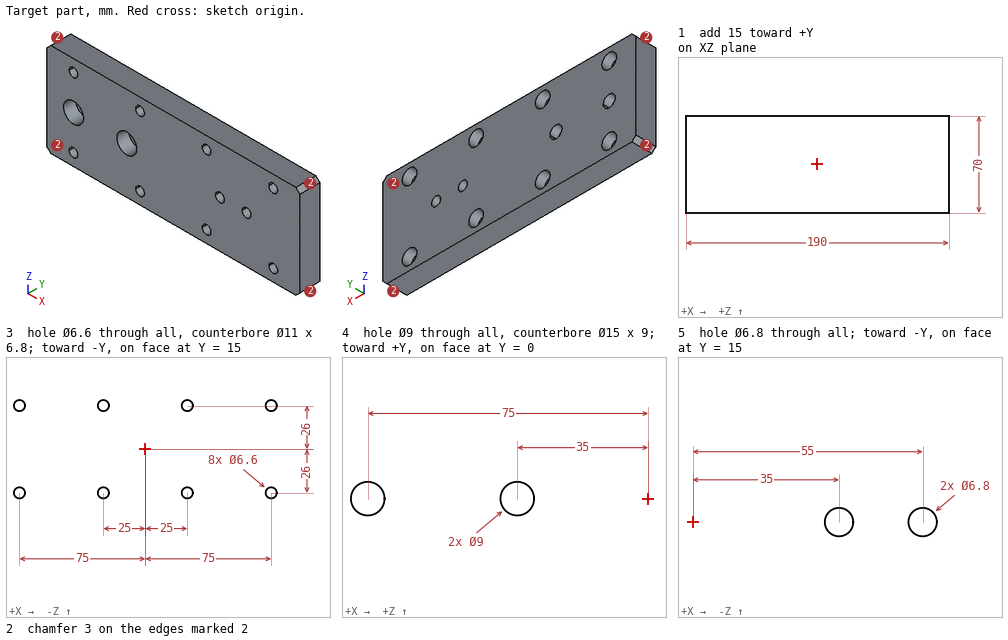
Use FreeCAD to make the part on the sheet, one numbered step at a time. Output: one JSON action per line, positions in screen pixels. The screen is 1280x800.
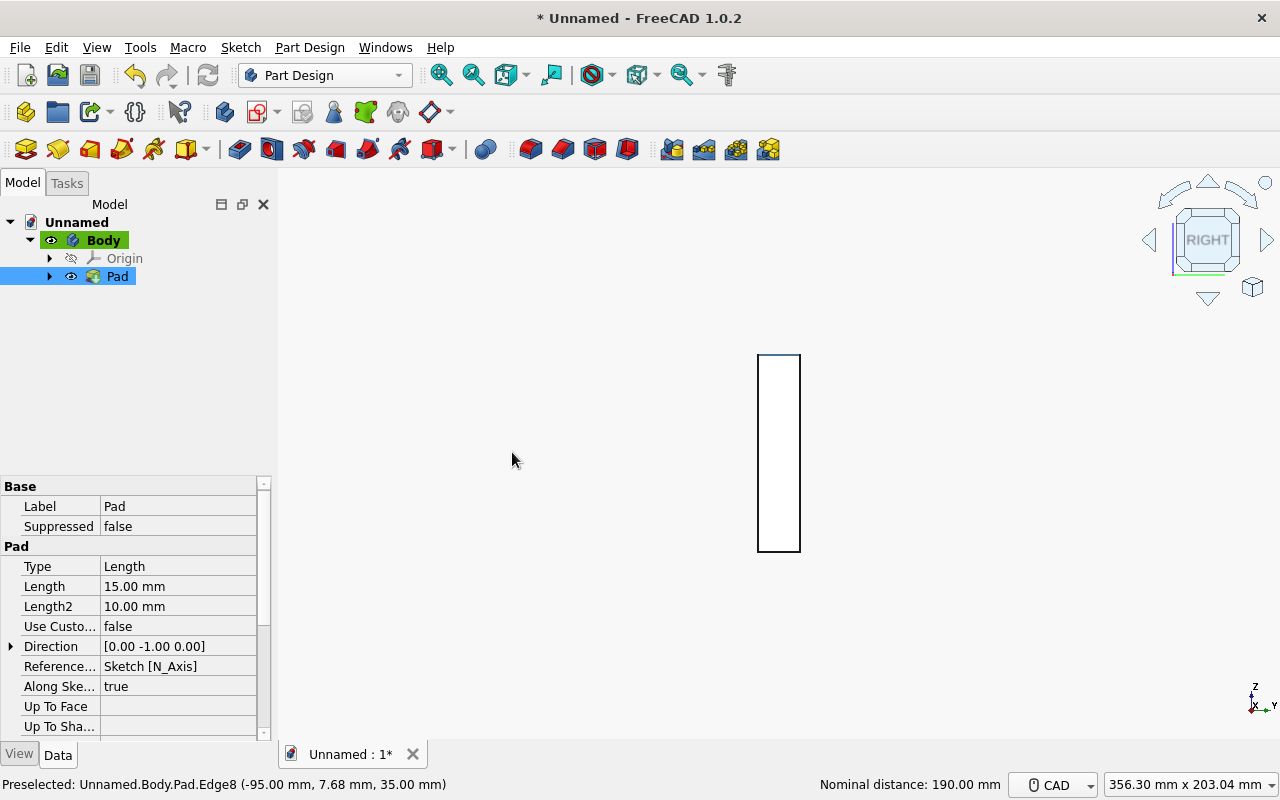
{"action": "key", "text": "v f"}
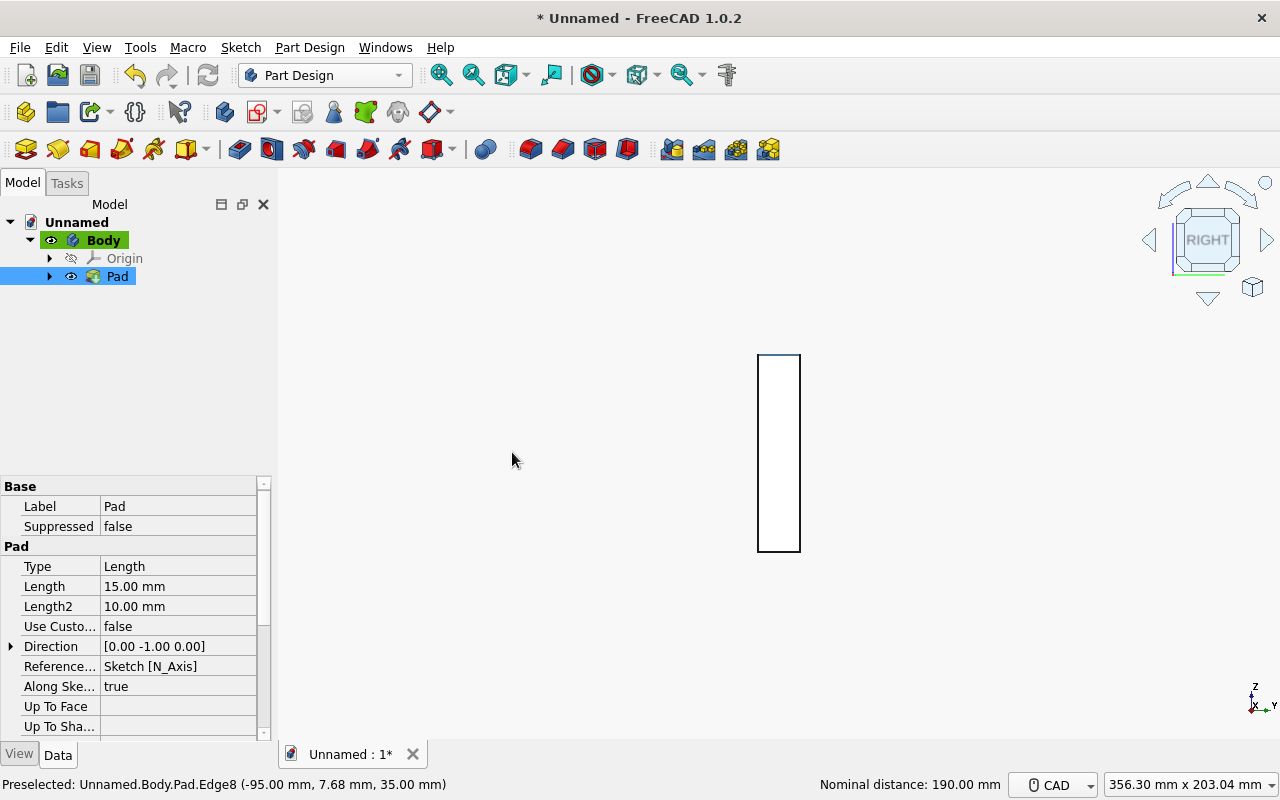
{"action": "left_click", "coordinate": [779, 551], "text": "ctrl"}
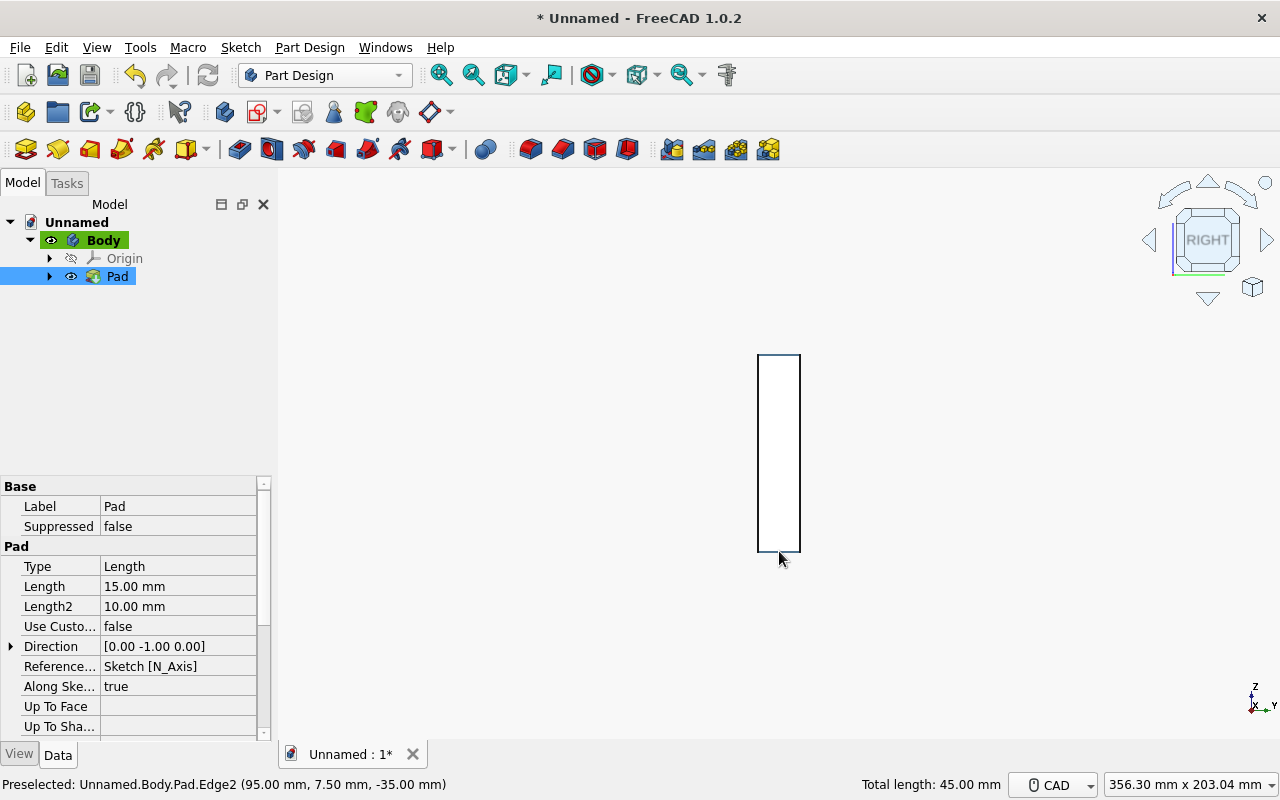
{"action": "key", "text": "5"}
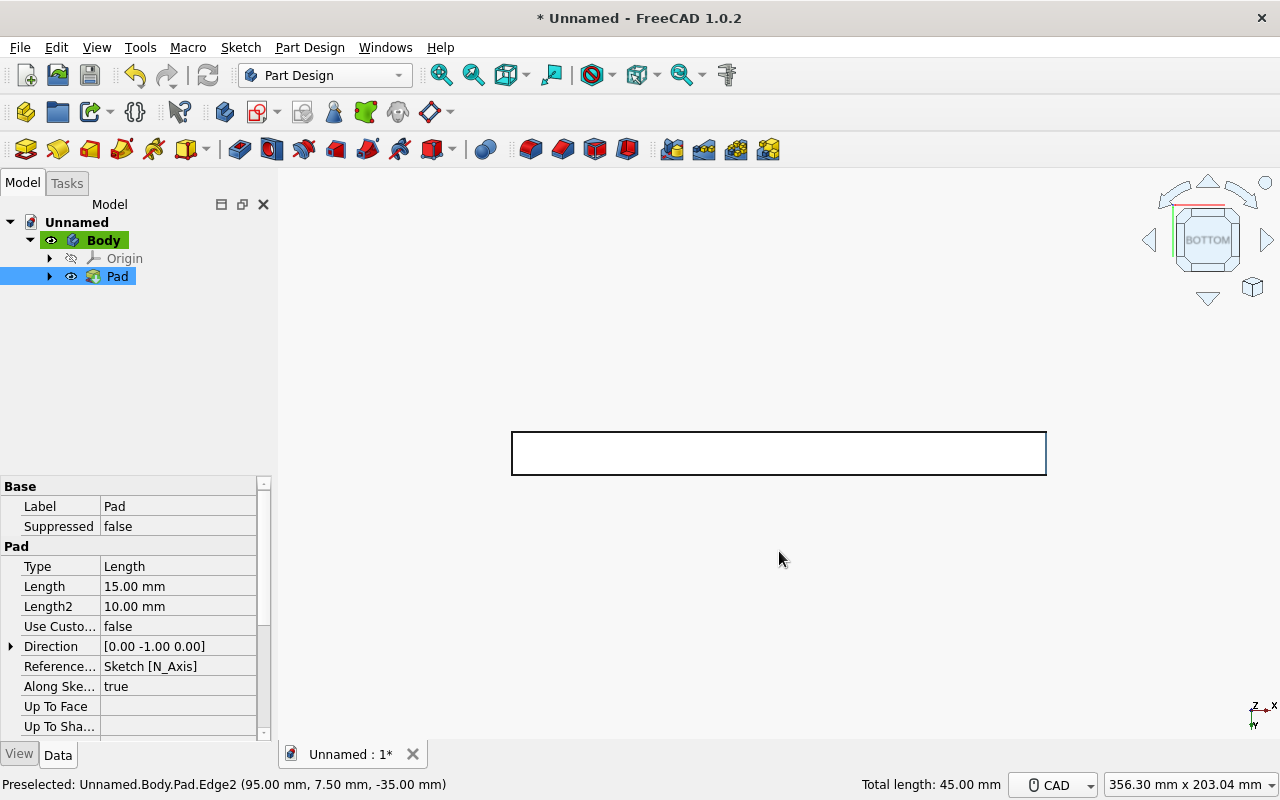
{"action": "left_click", "coordinate": [512, 452], "text": "ctrl"}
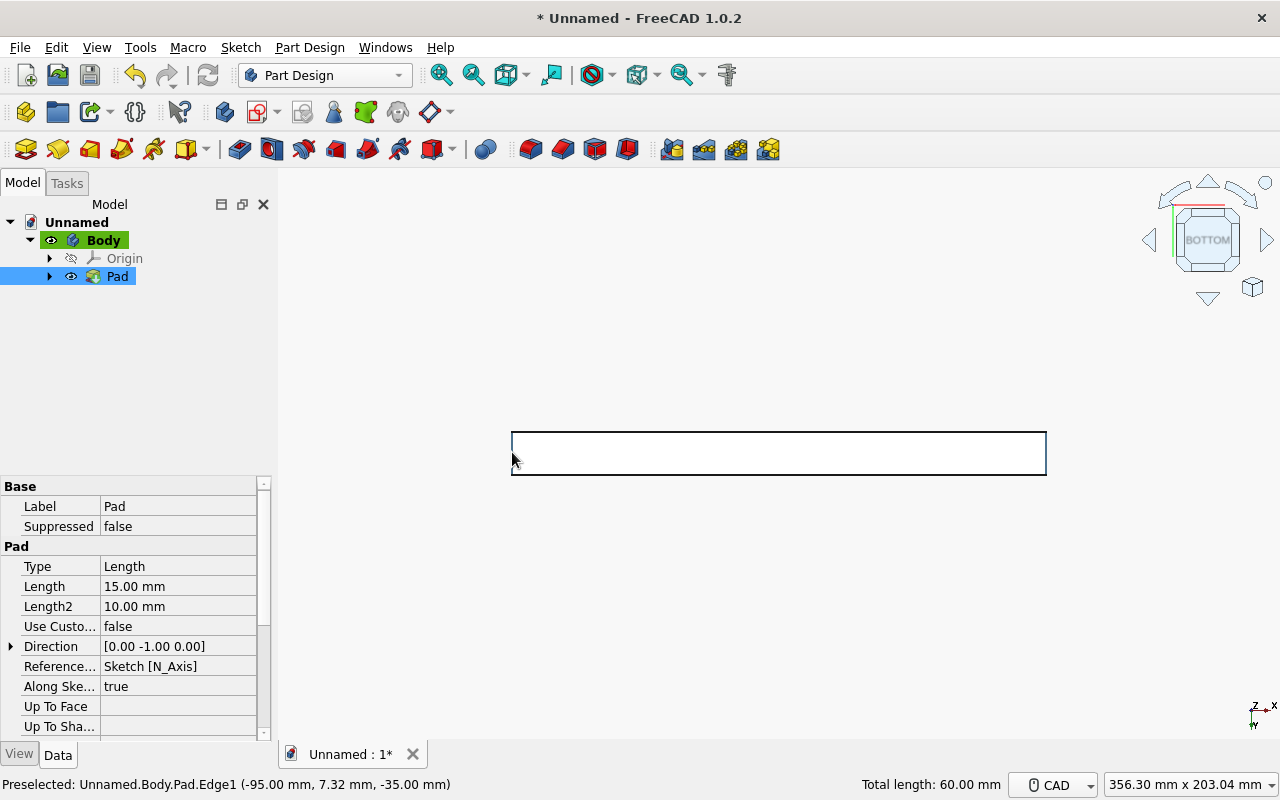
{"action": "left_click", "coordinate": [564, 150]}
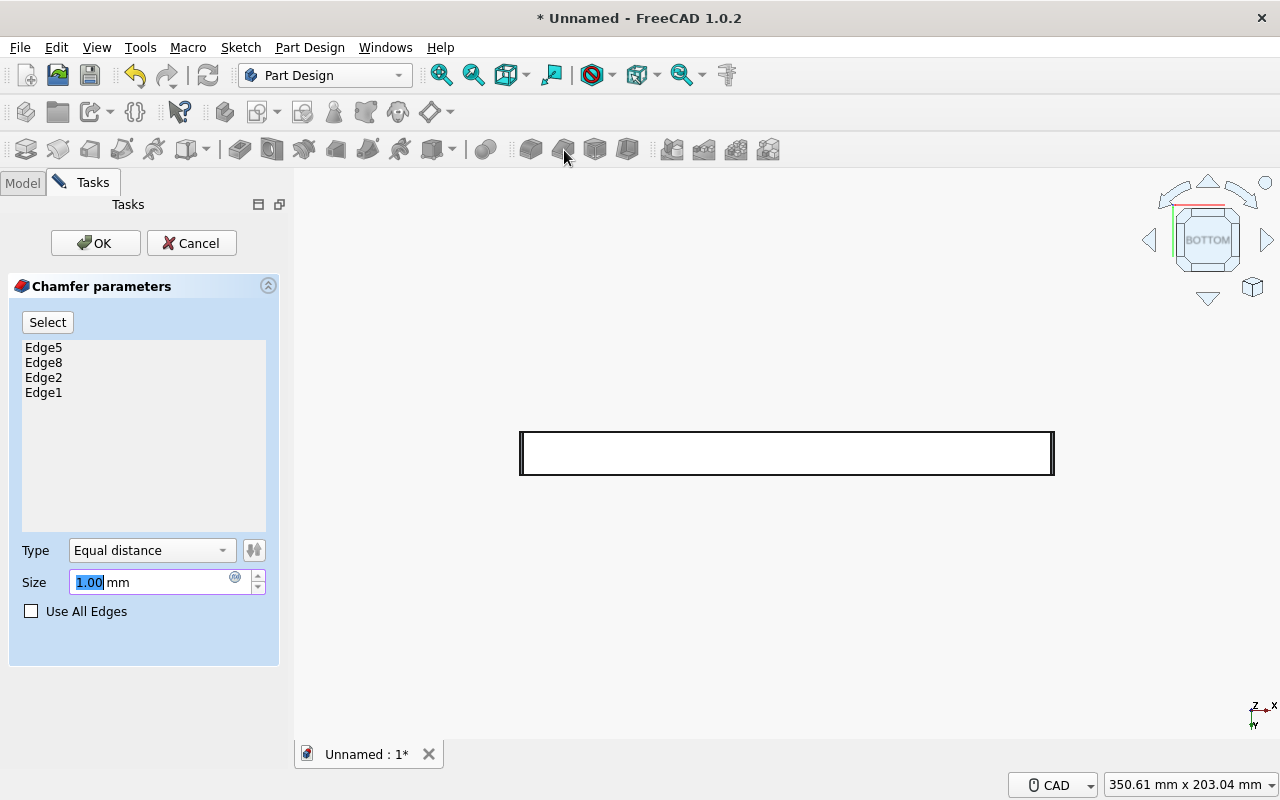
{"action": "type", "text": "3"}
{"action": "key", "text": "Tab"}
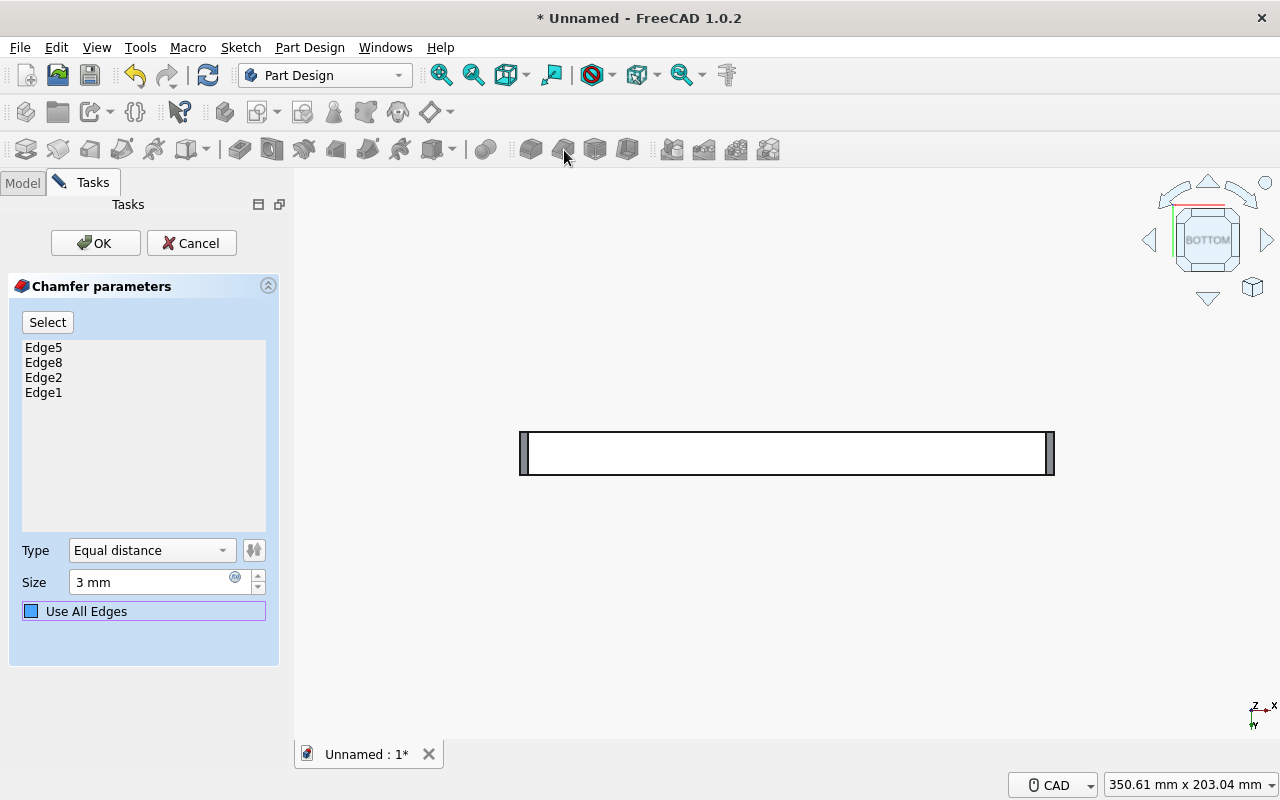
{"action": "left_click", "coordinate": [96, 243]}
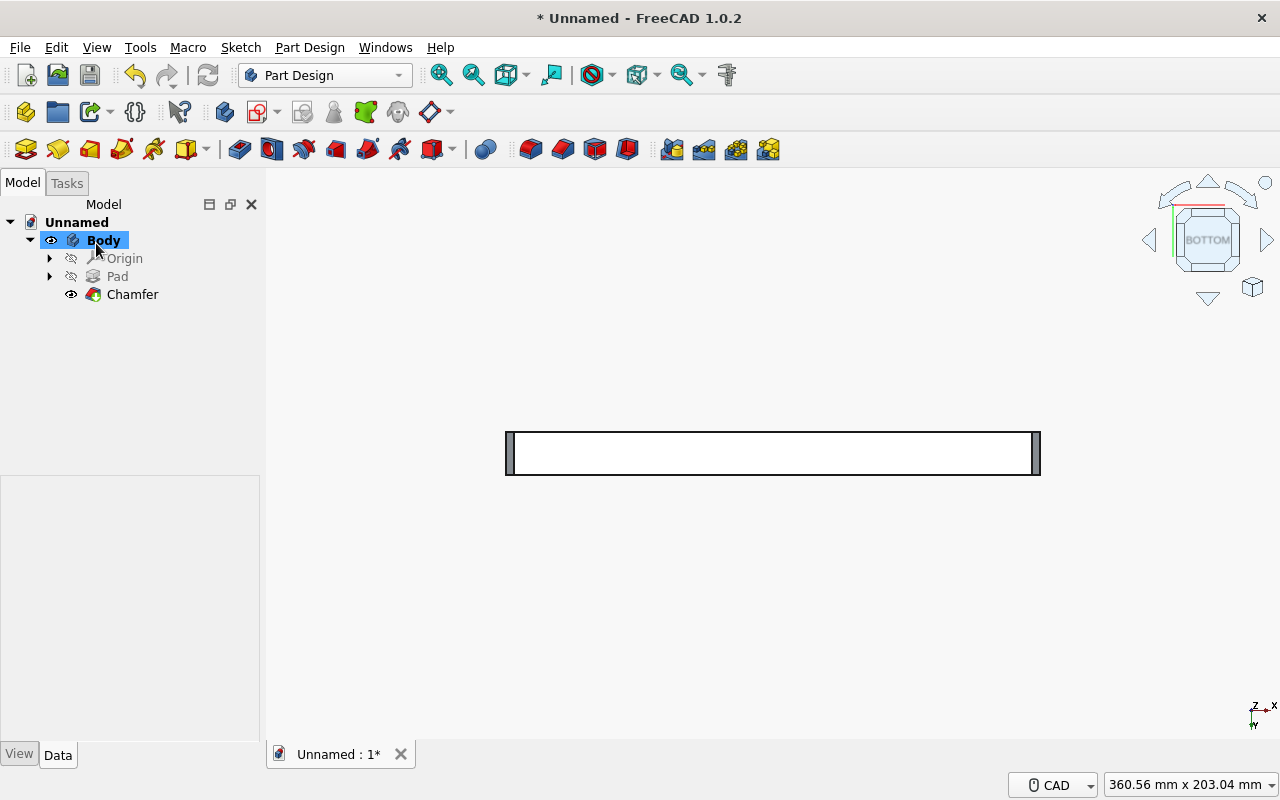
{"action": "key", "text": "4"}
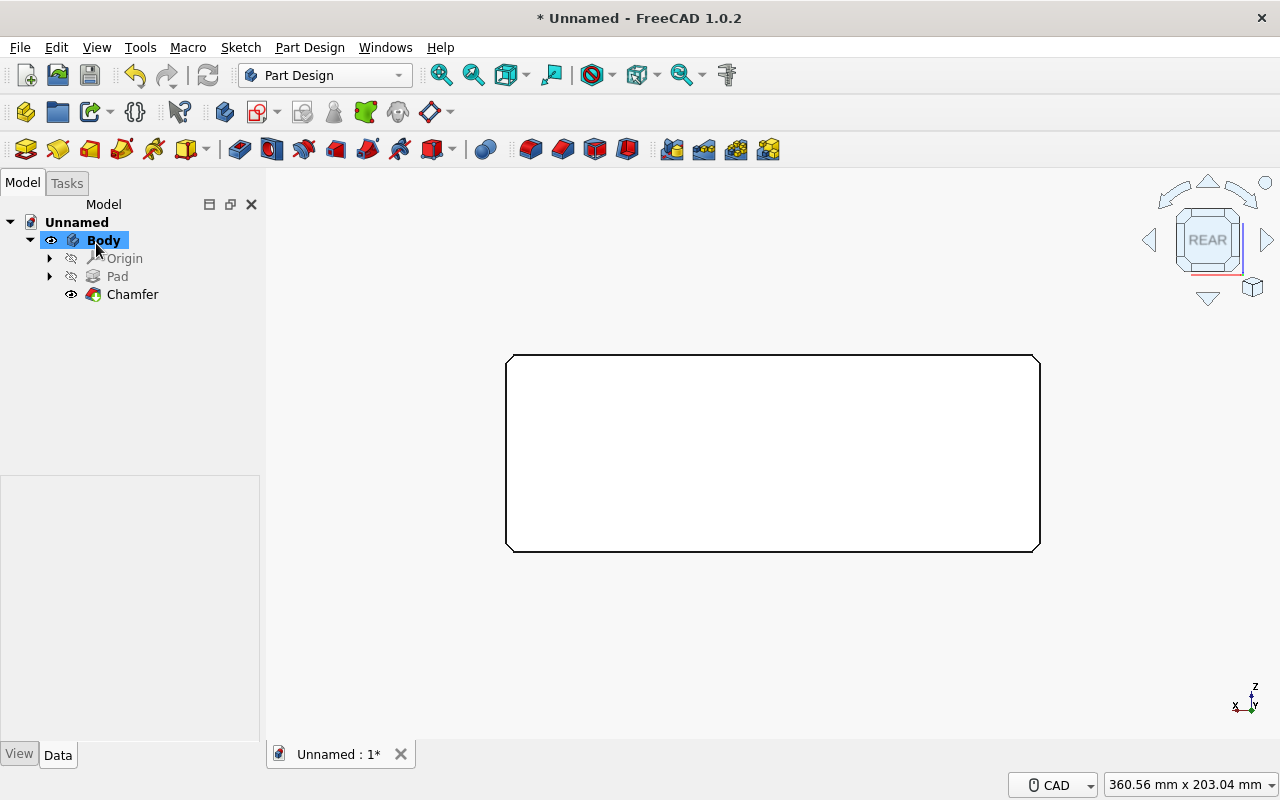
{"action": "left_click", "coordinate": [620, 453]}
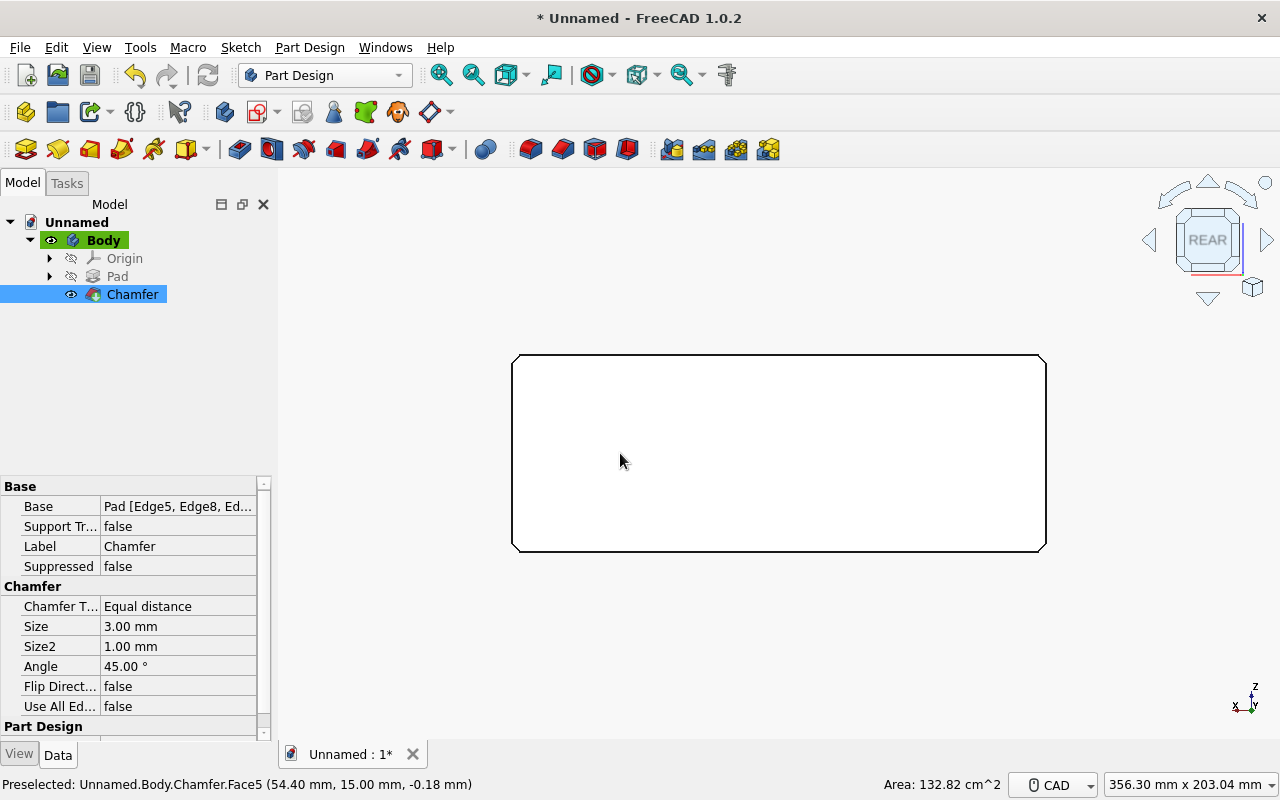
{"action": "left_click", "coordinate": [258, 112]}